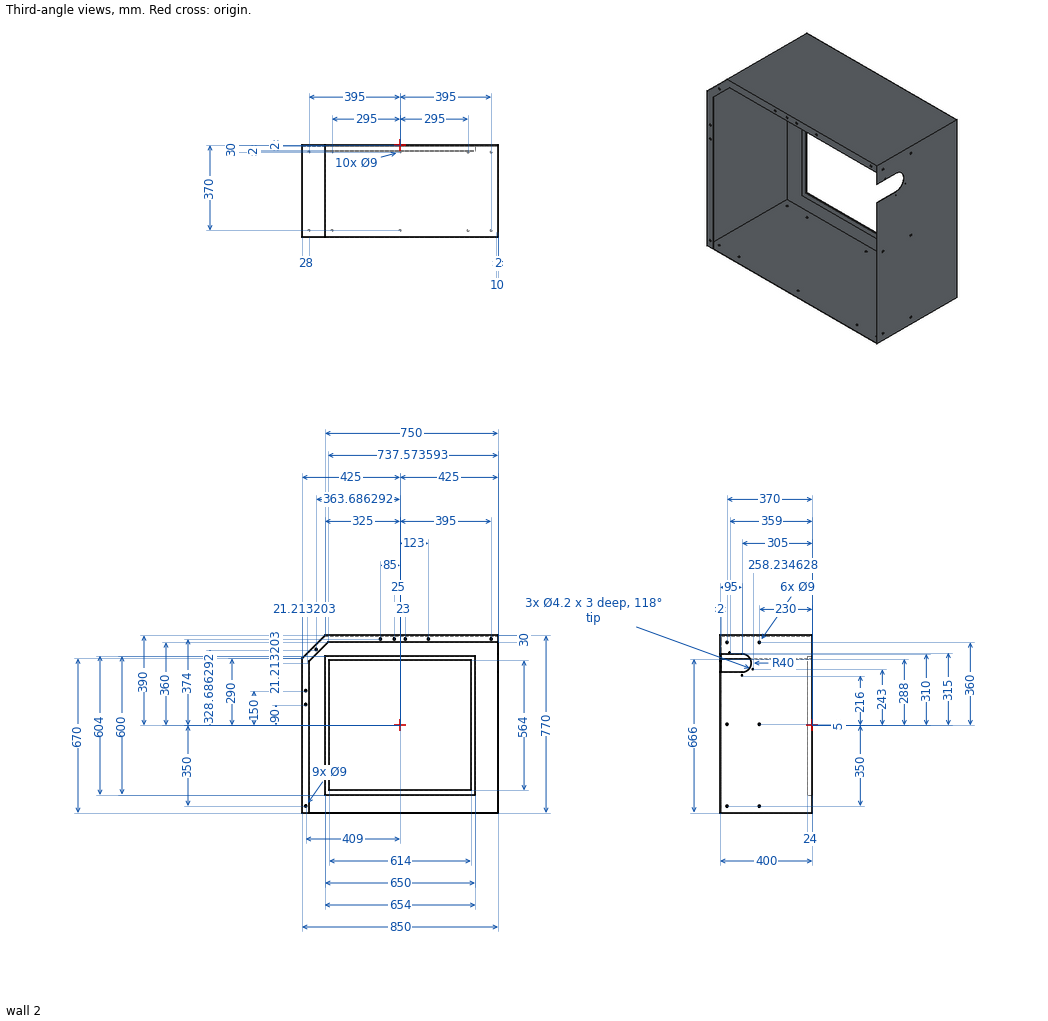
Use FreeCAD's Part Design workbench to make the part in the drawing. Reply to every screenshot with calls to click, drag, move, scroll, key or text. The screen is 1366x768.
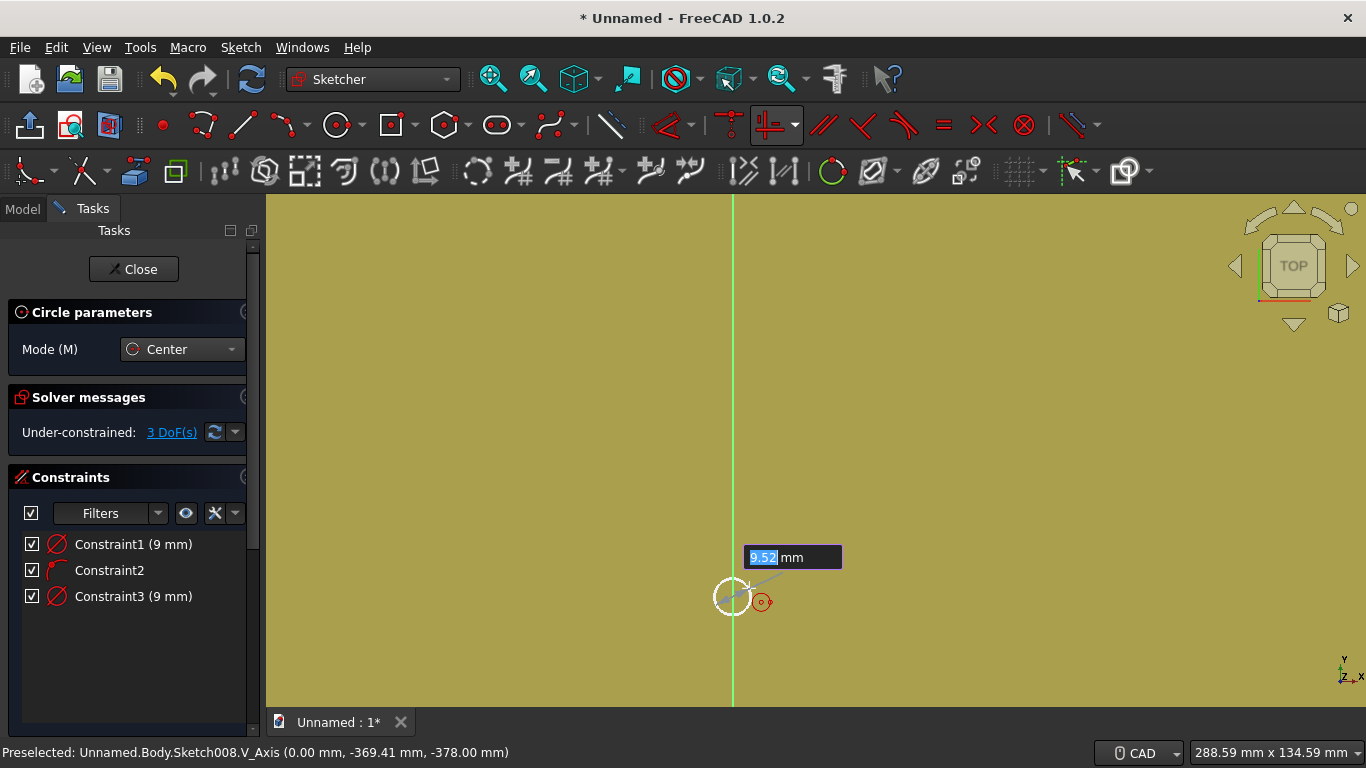
text(9)
key(Return)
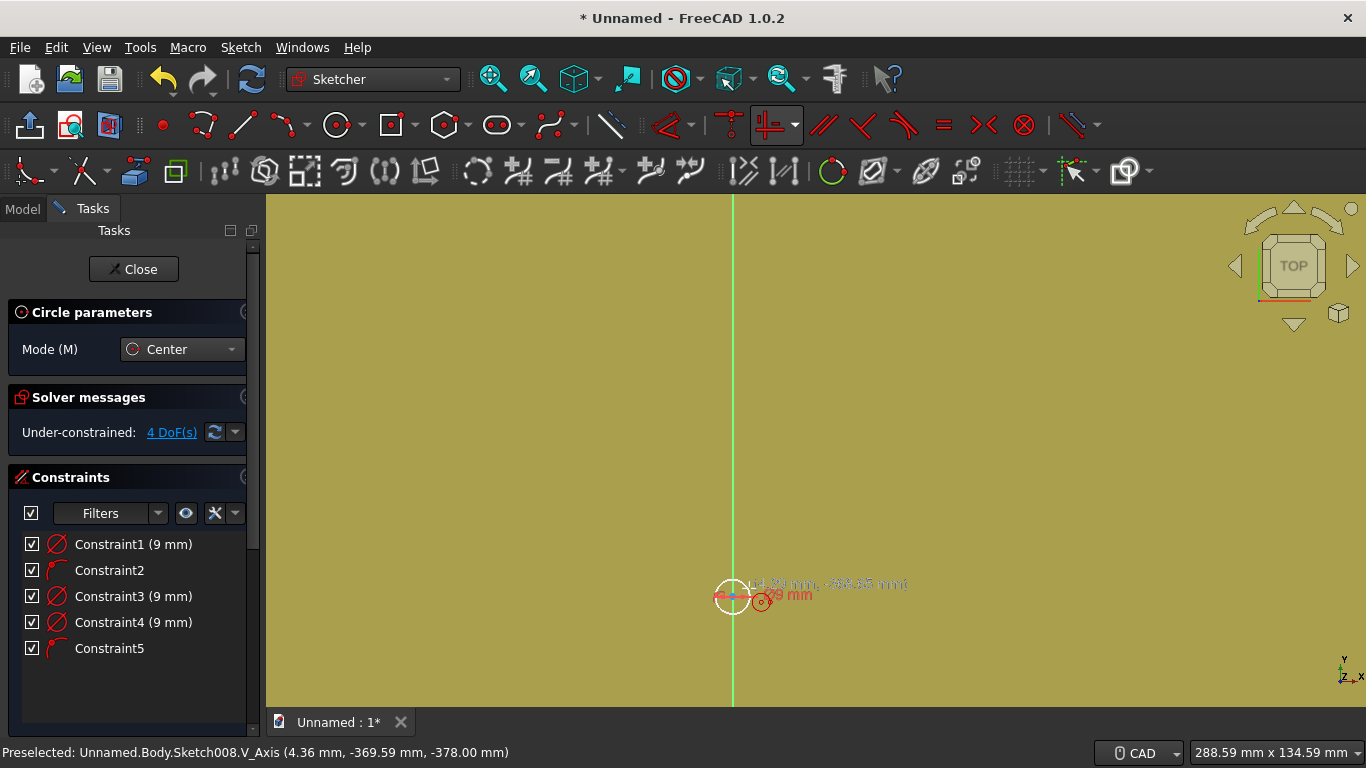
scroll(751, 590, down, 8)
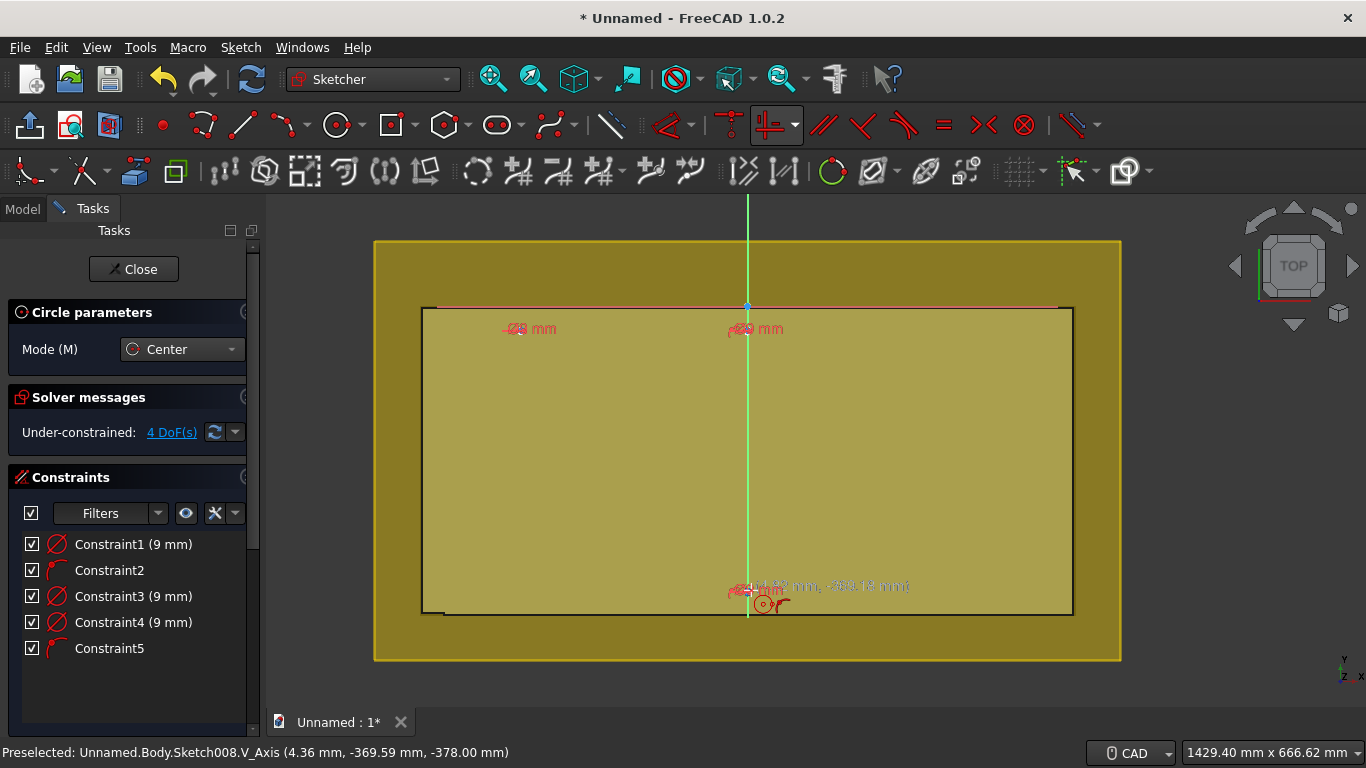
scroll(521, 591, up, 10)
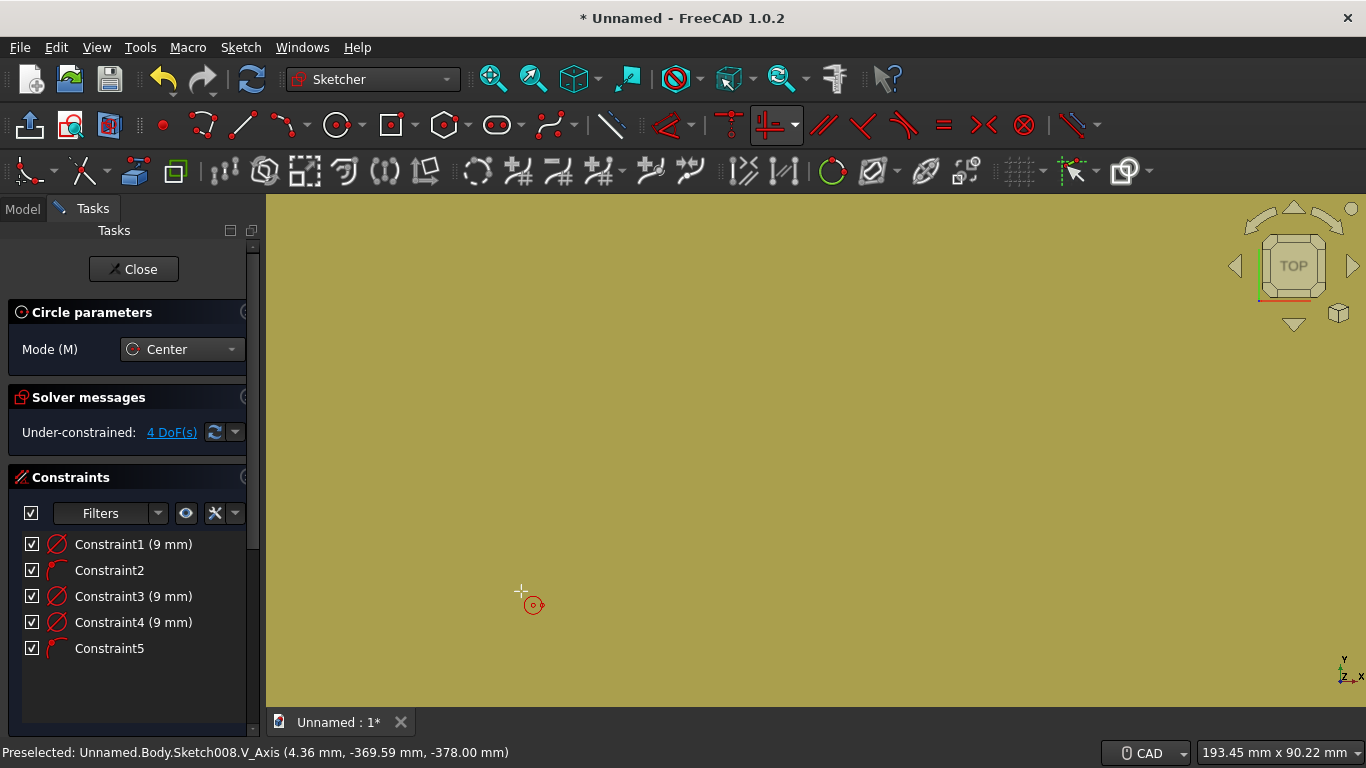
scroll(521, 591, down, 10)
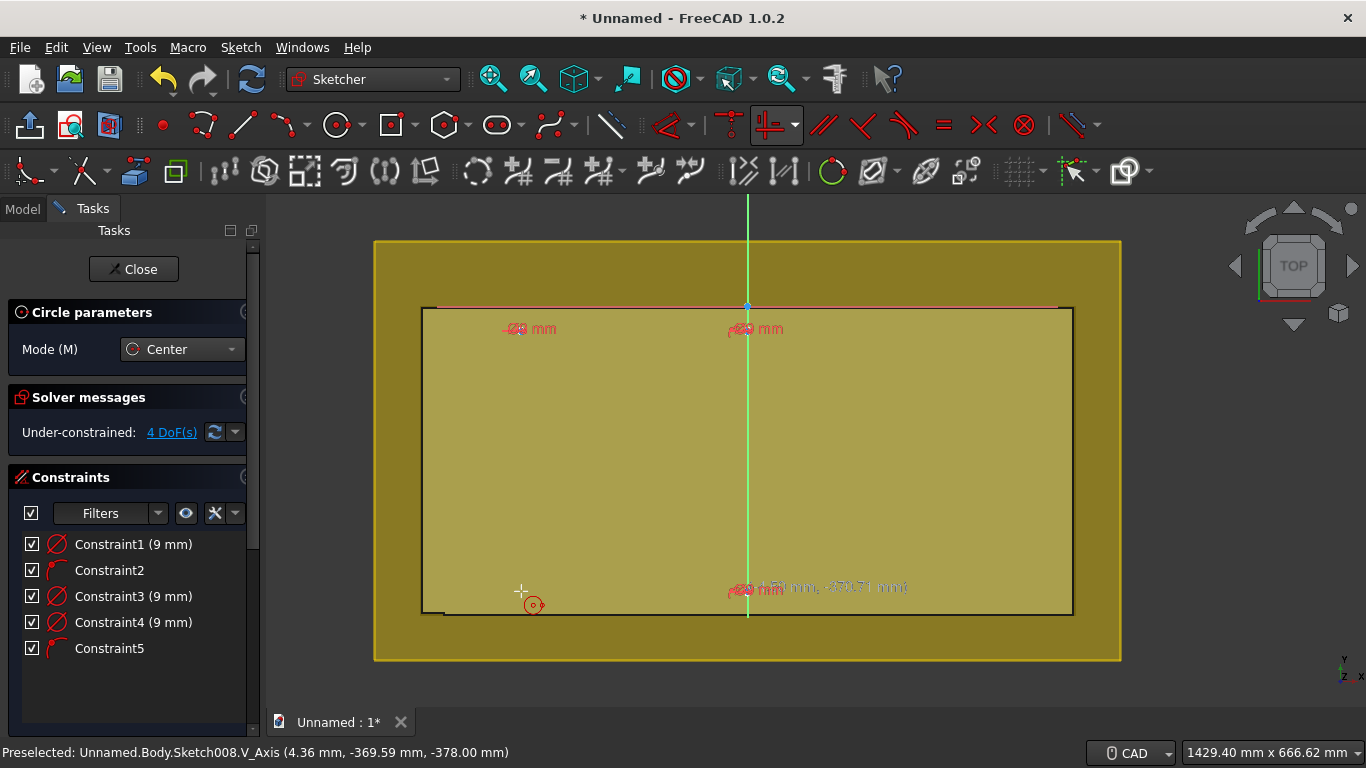
click(521, 591)
move(523, 589)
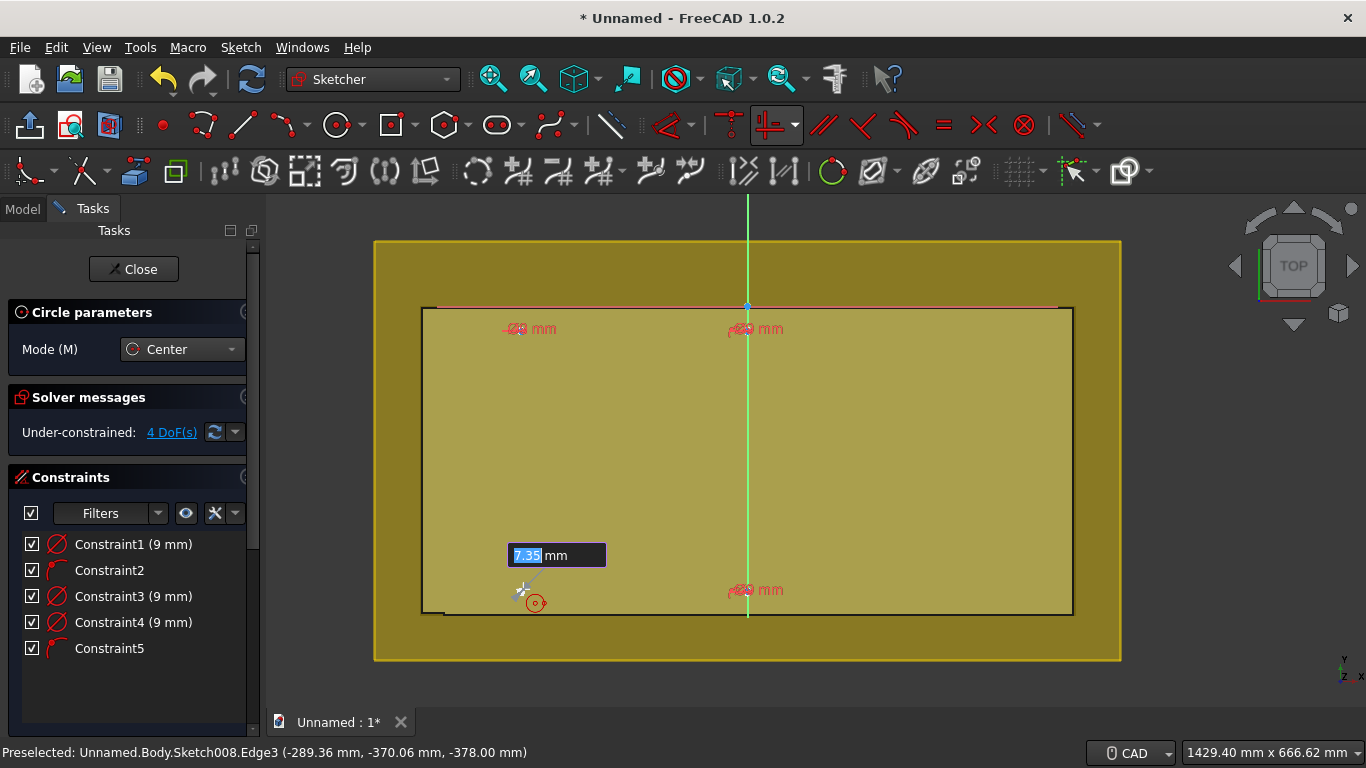
text(9)
key(Return)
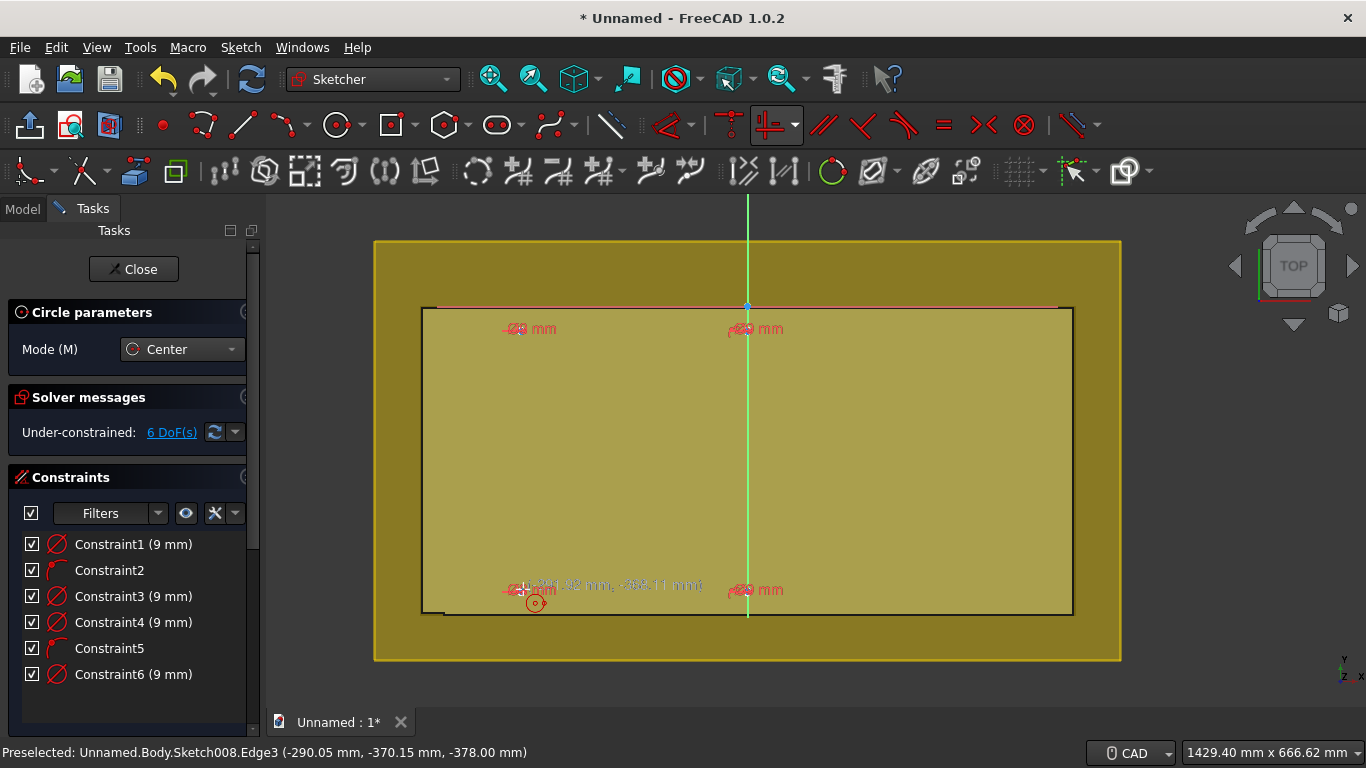
scroll(444, 330, up, 10)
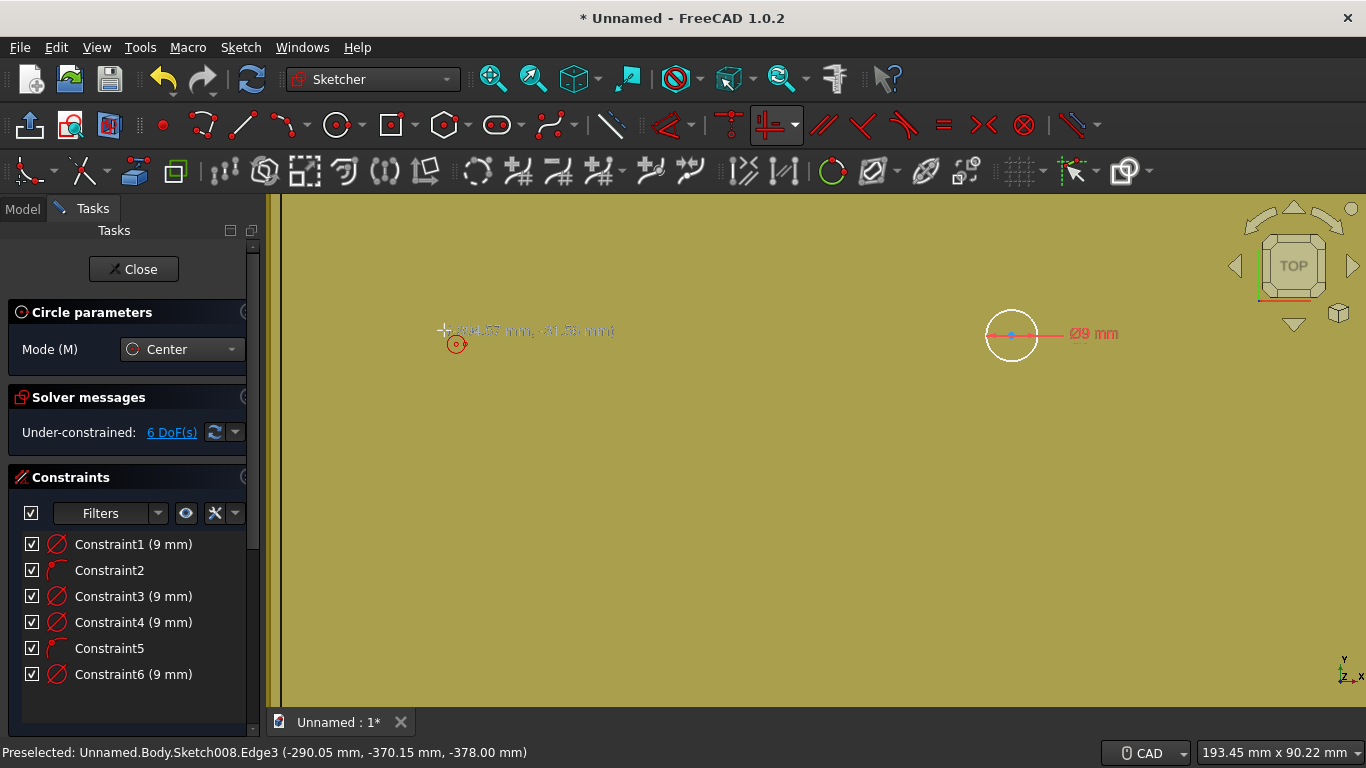
scroll(444, 330, down, 10)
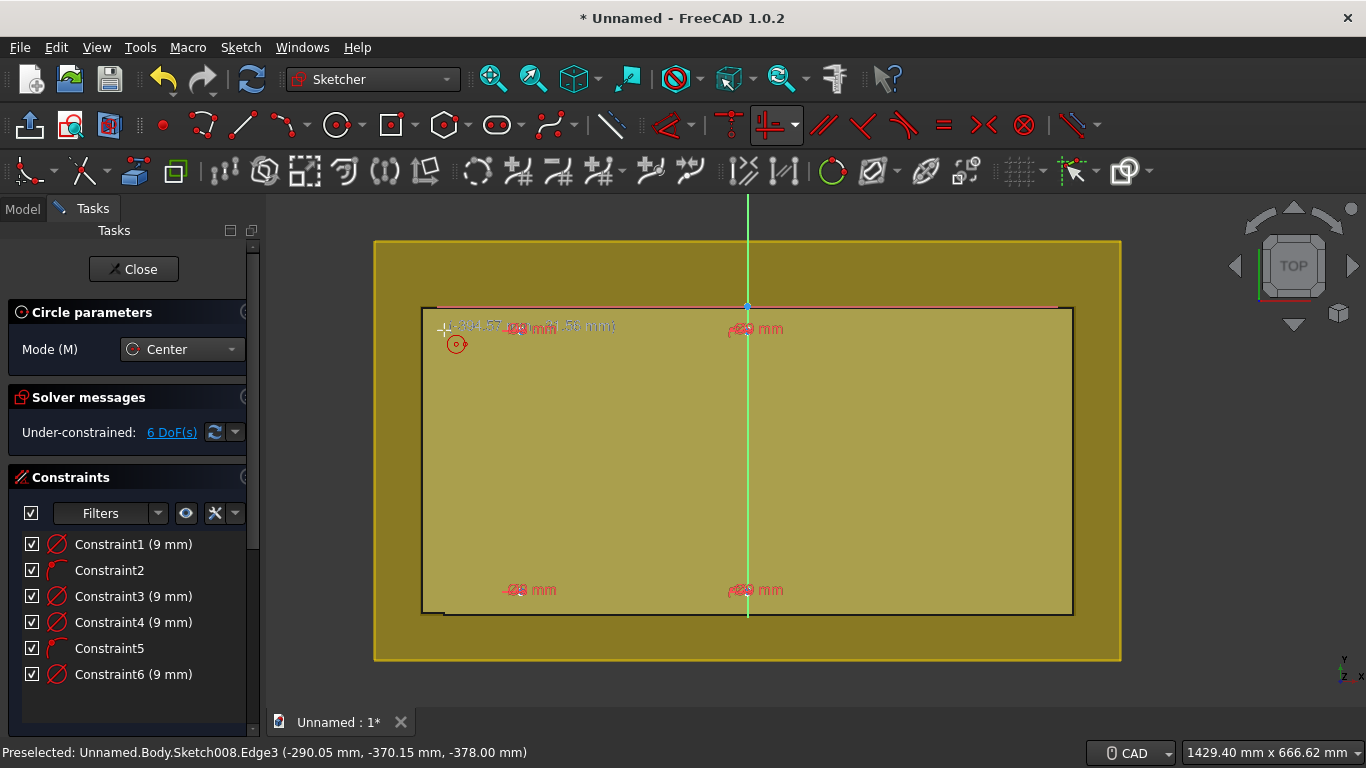
click(444, 330)
move(446, 327)